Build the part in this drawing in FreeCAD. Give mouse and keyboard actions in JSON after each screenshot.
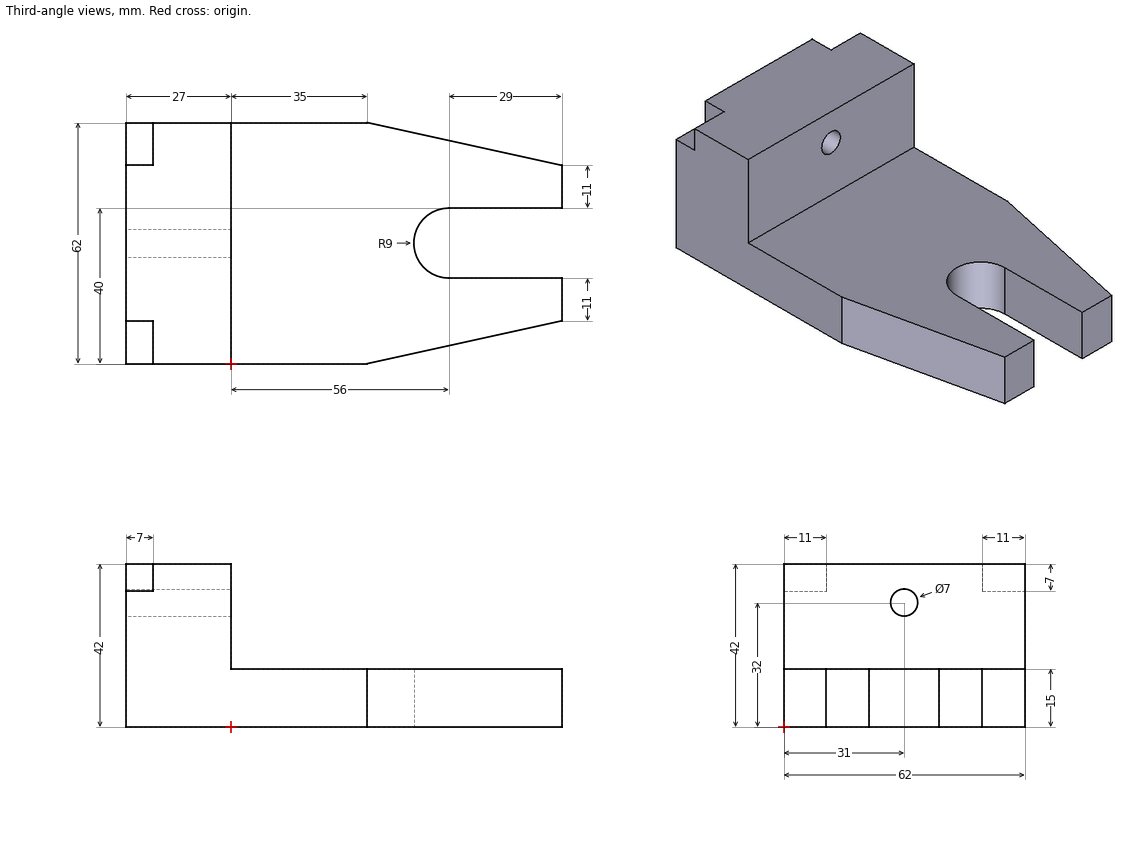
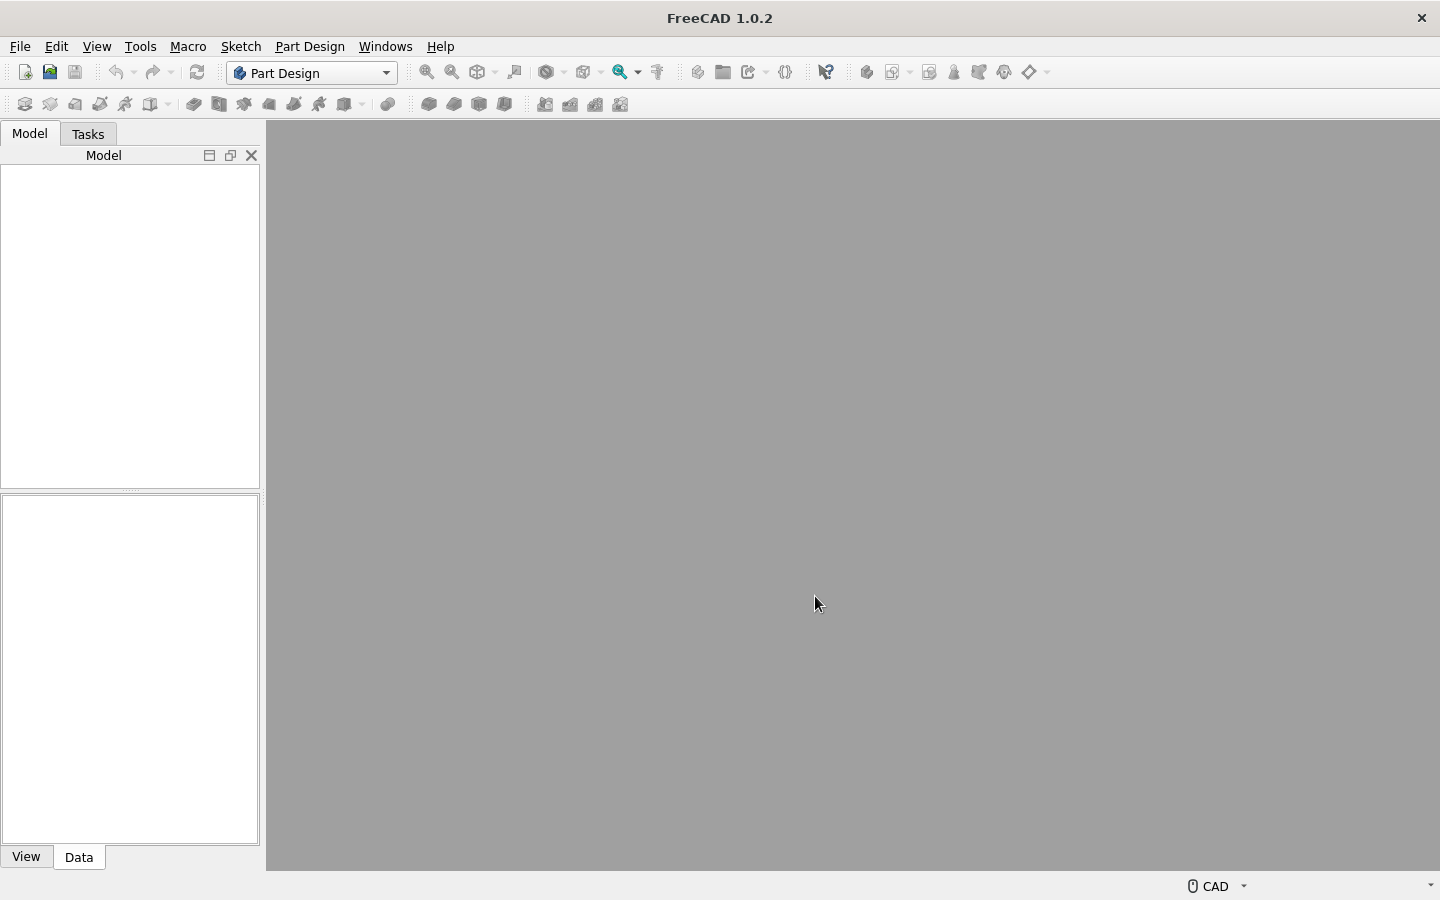
{"action": "left_click", "coordinate": [25, 72]}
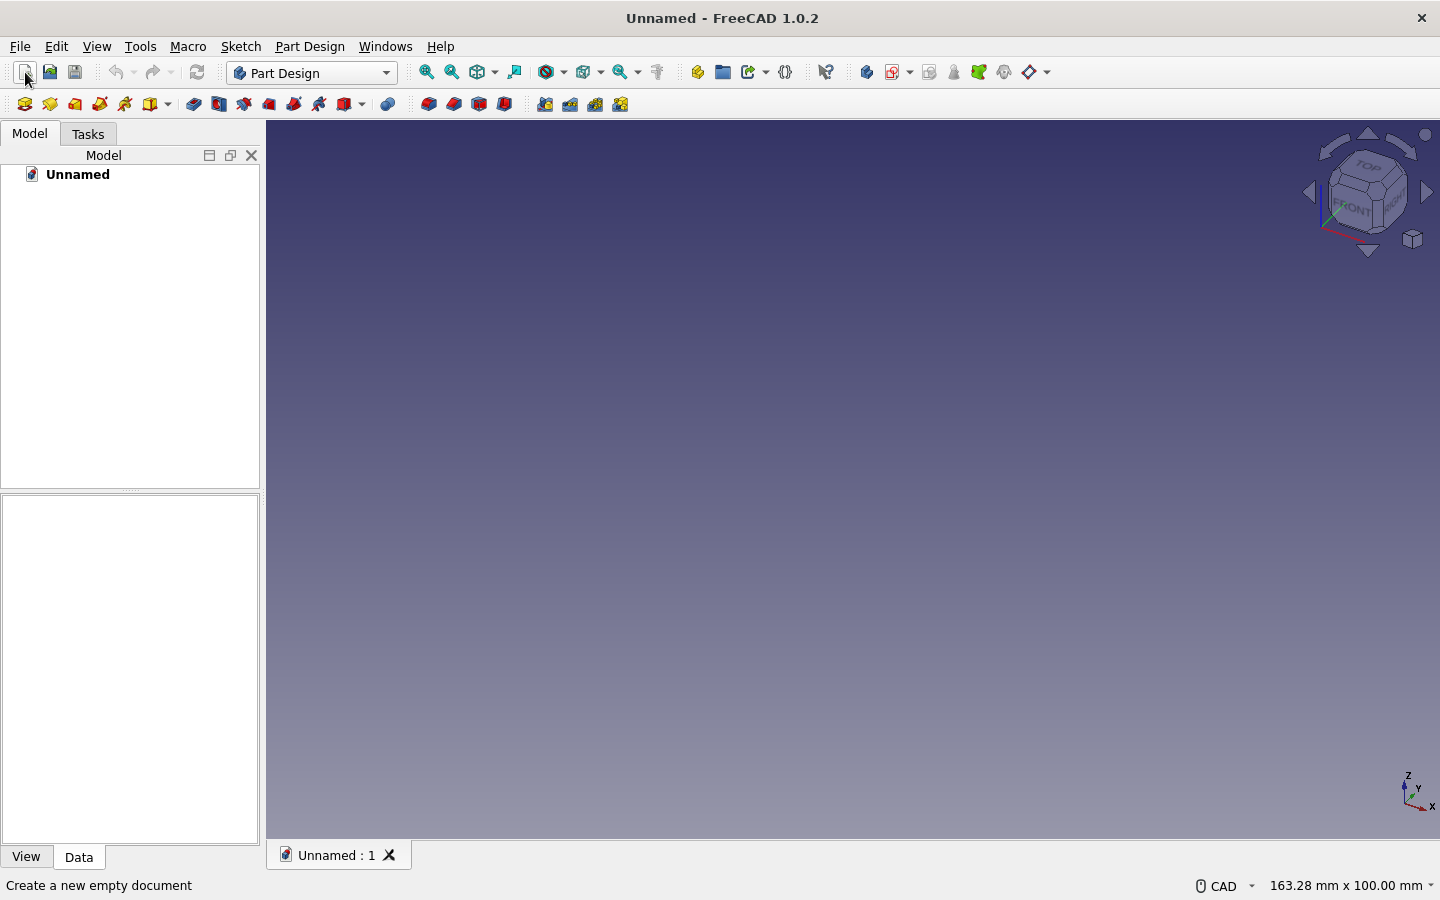
{"action": "left_click", "coordinate": [892, 72]}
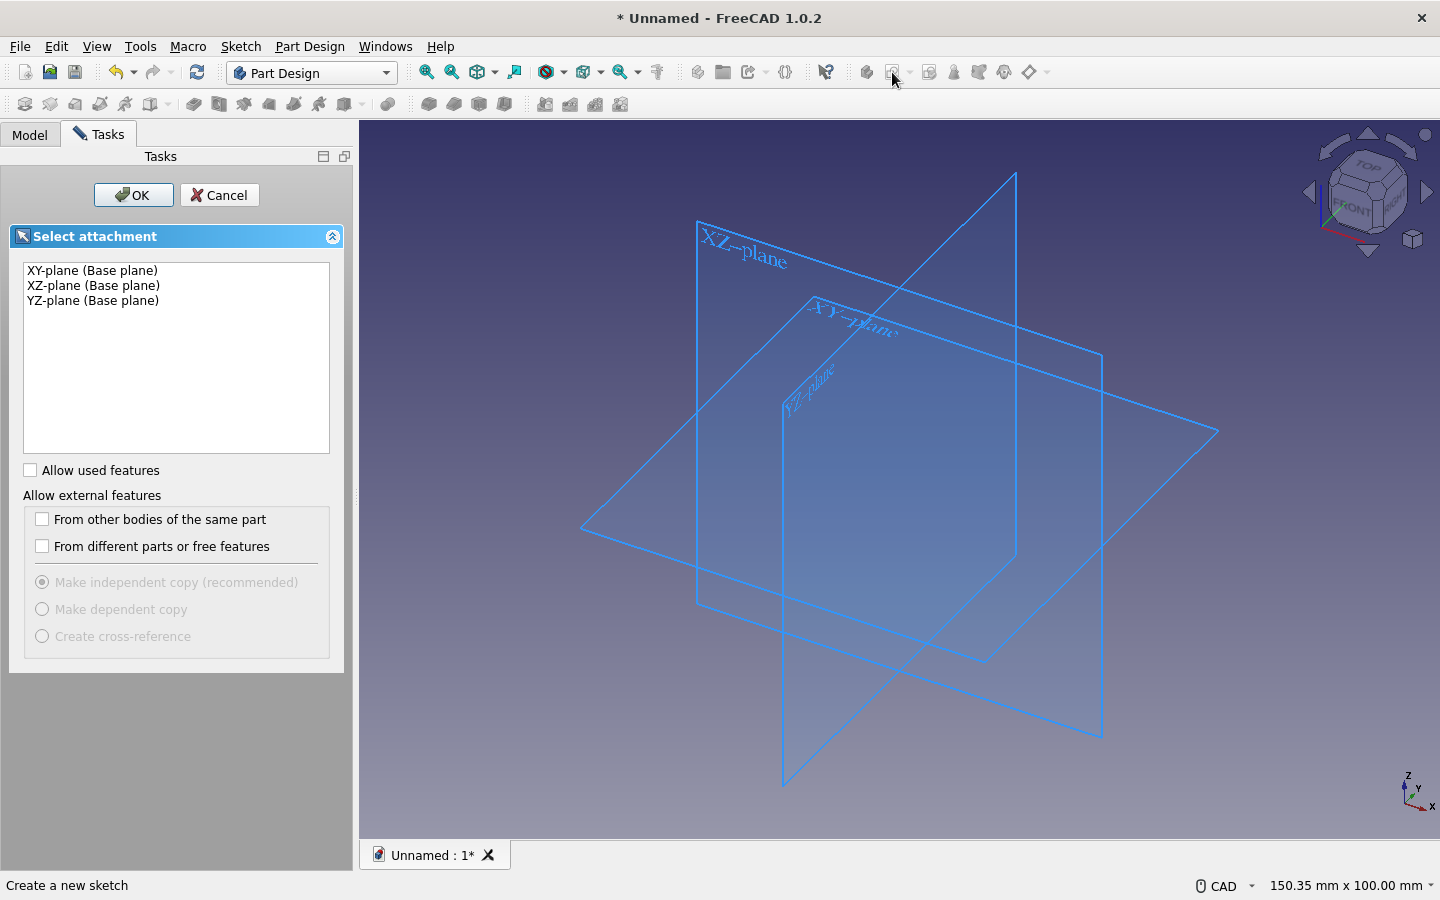
{"action": "left_click", "coordinate": [84, 270]}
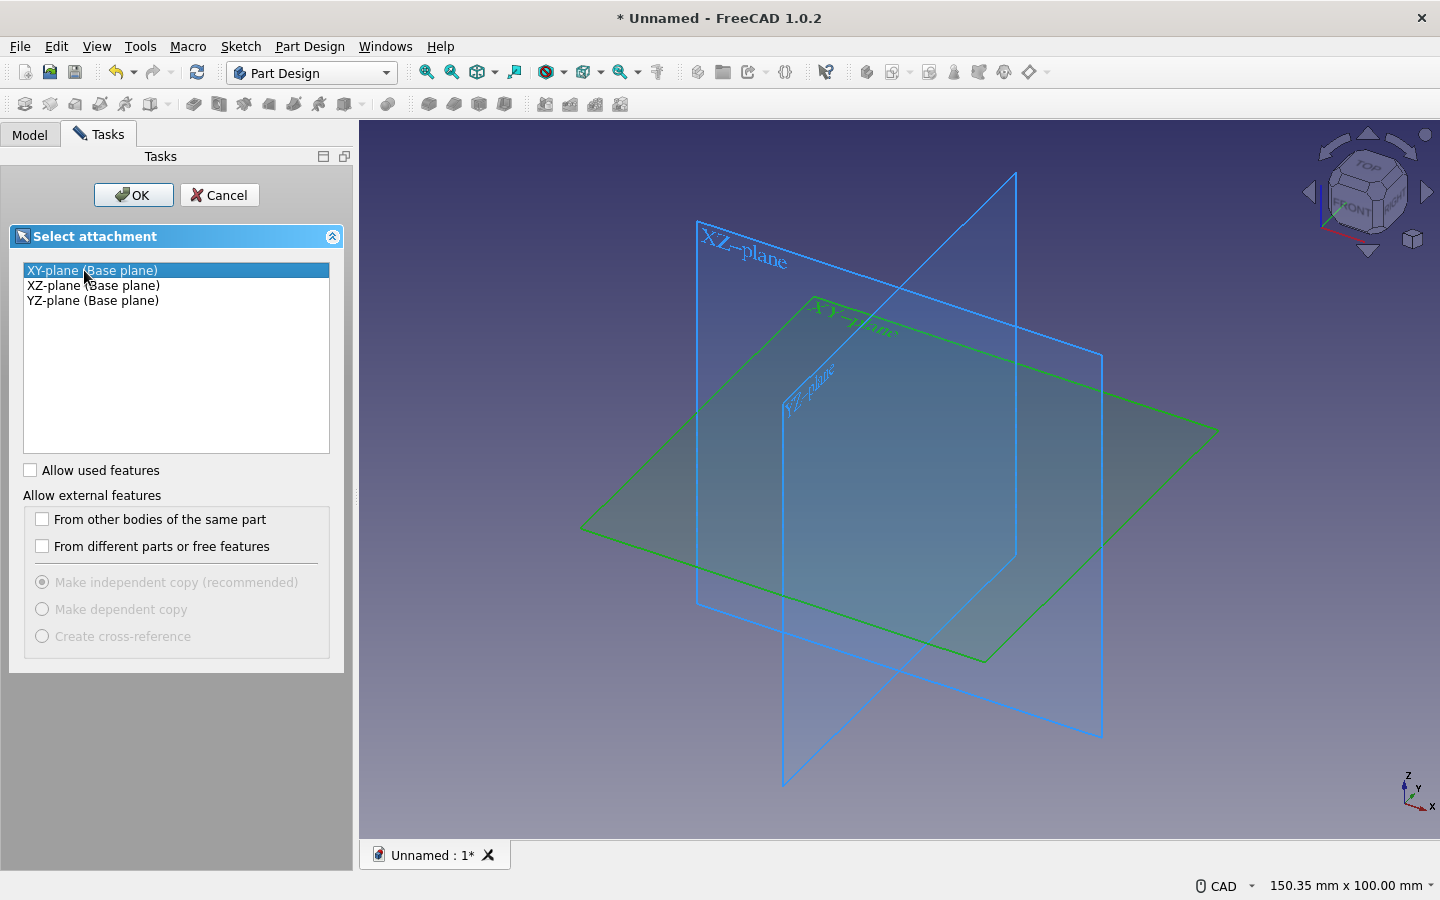
{"action": "left_click", "coordinate": [134, 195]}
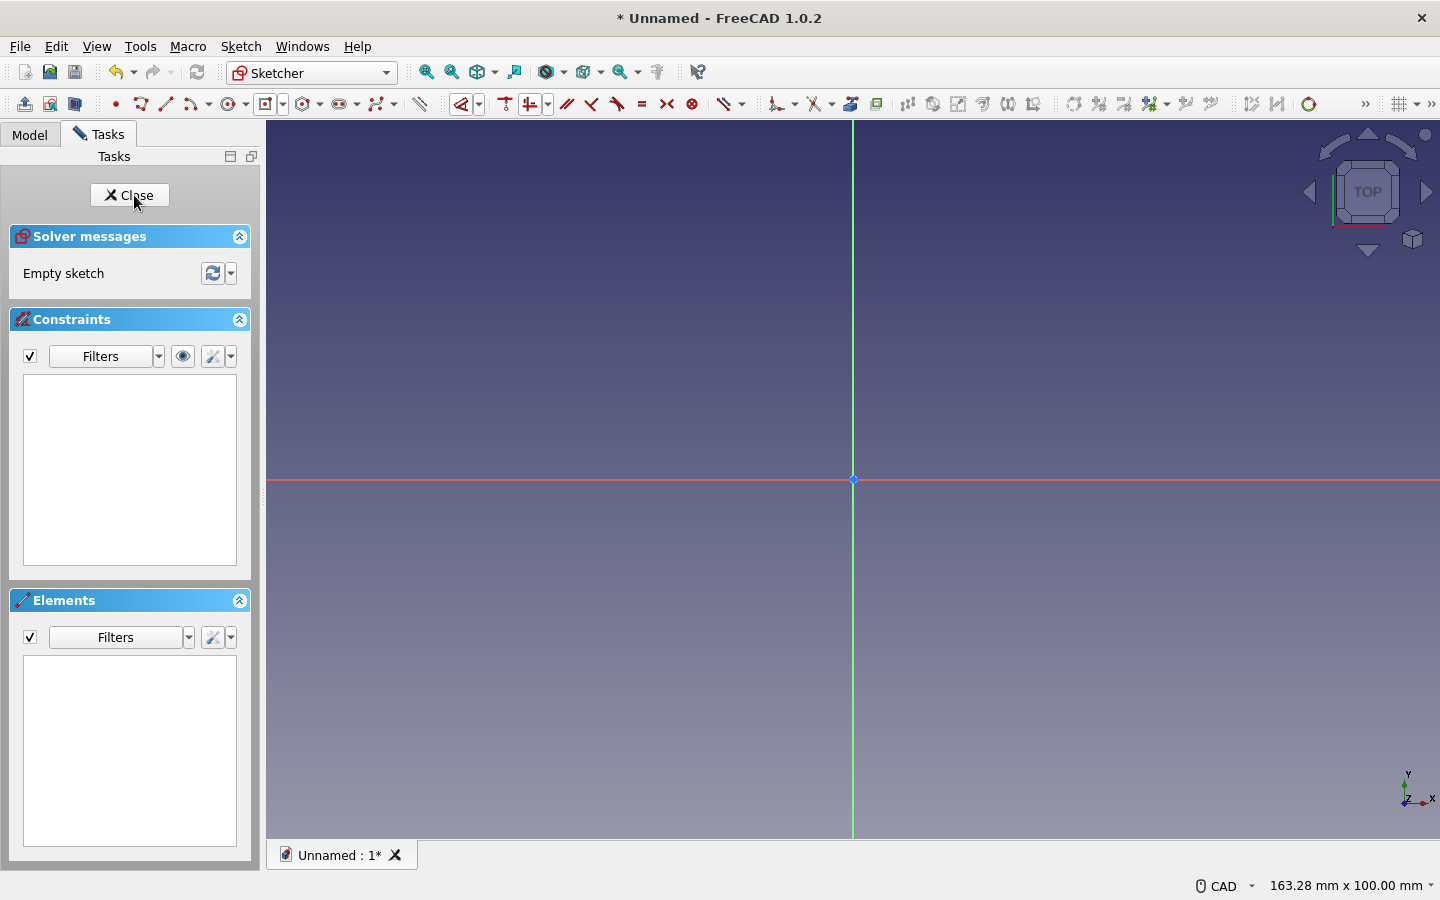
{"action": "scroll", "coordinate": [294, 811], "scroll_direction": "down", "scroll_amount": 2}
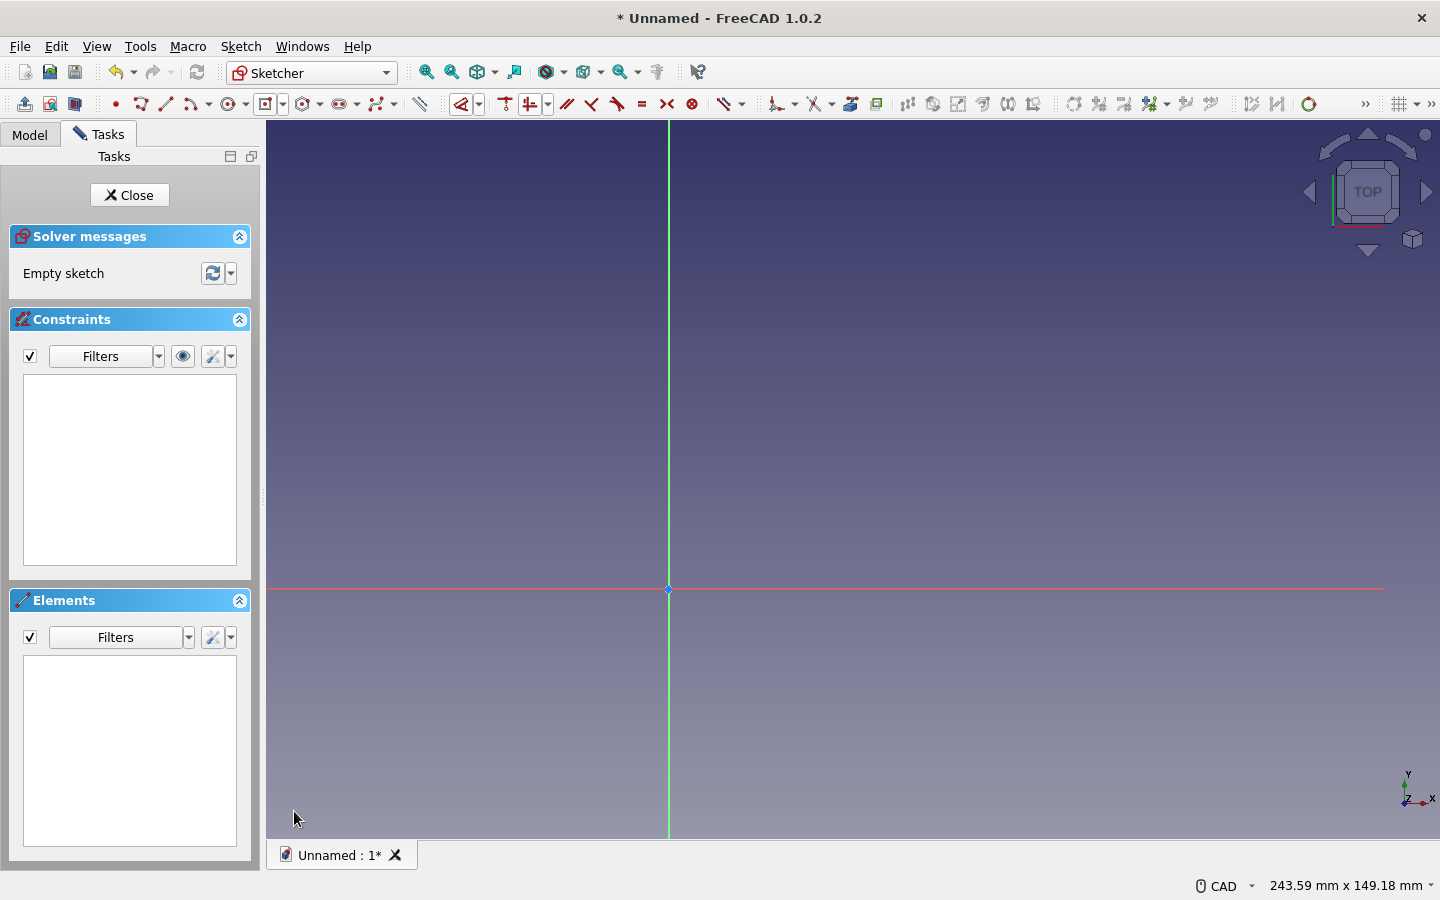
{"action": "scroll", "coordinate": [1055, 359], "scroll_direction": "up", "scroll_amount": 2}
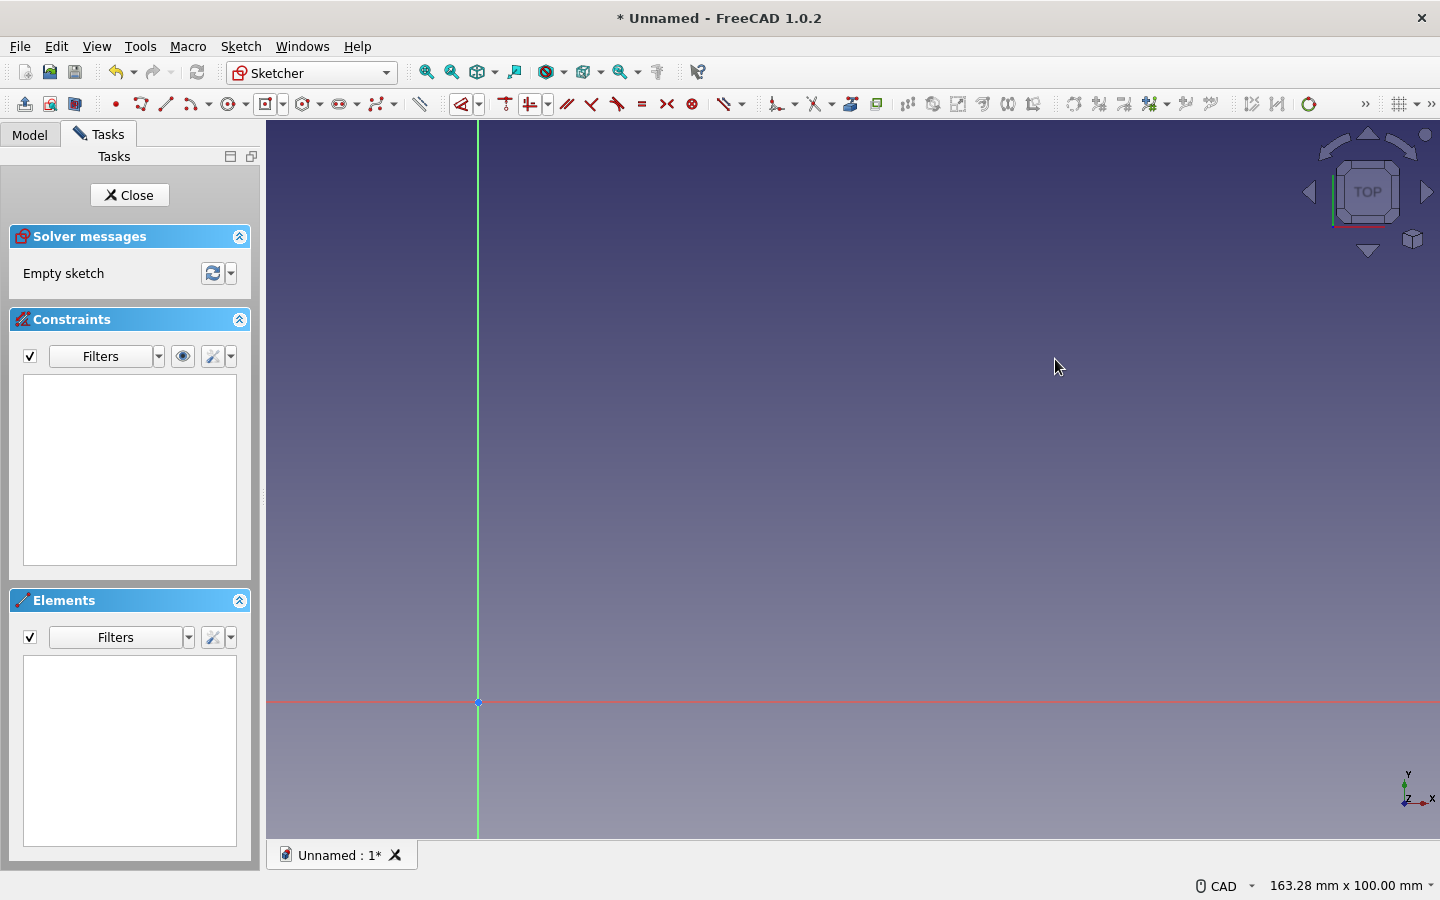
{"action": "left_click", "coordinate": [141, 104]}